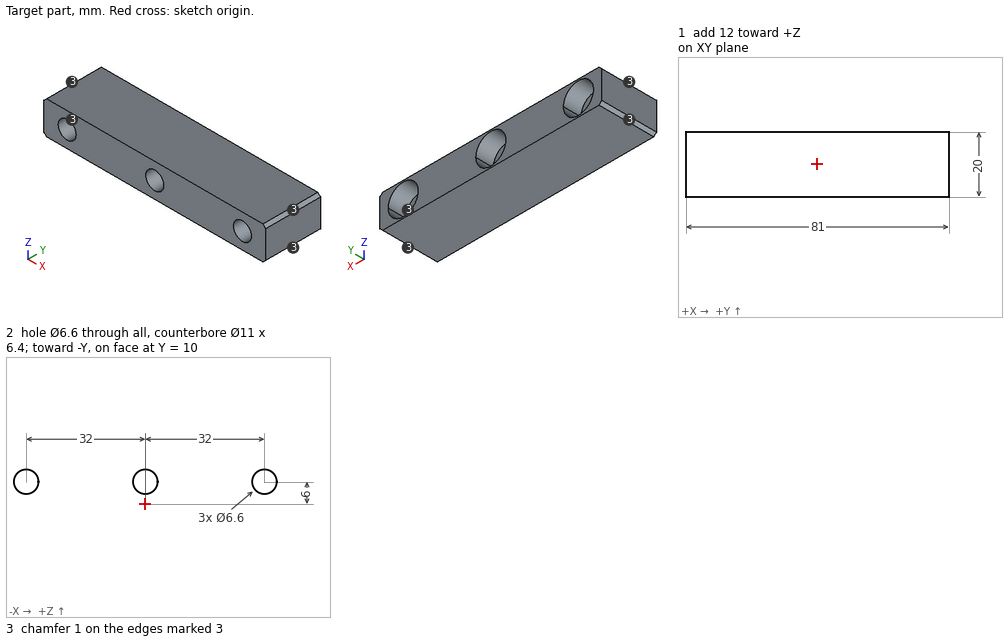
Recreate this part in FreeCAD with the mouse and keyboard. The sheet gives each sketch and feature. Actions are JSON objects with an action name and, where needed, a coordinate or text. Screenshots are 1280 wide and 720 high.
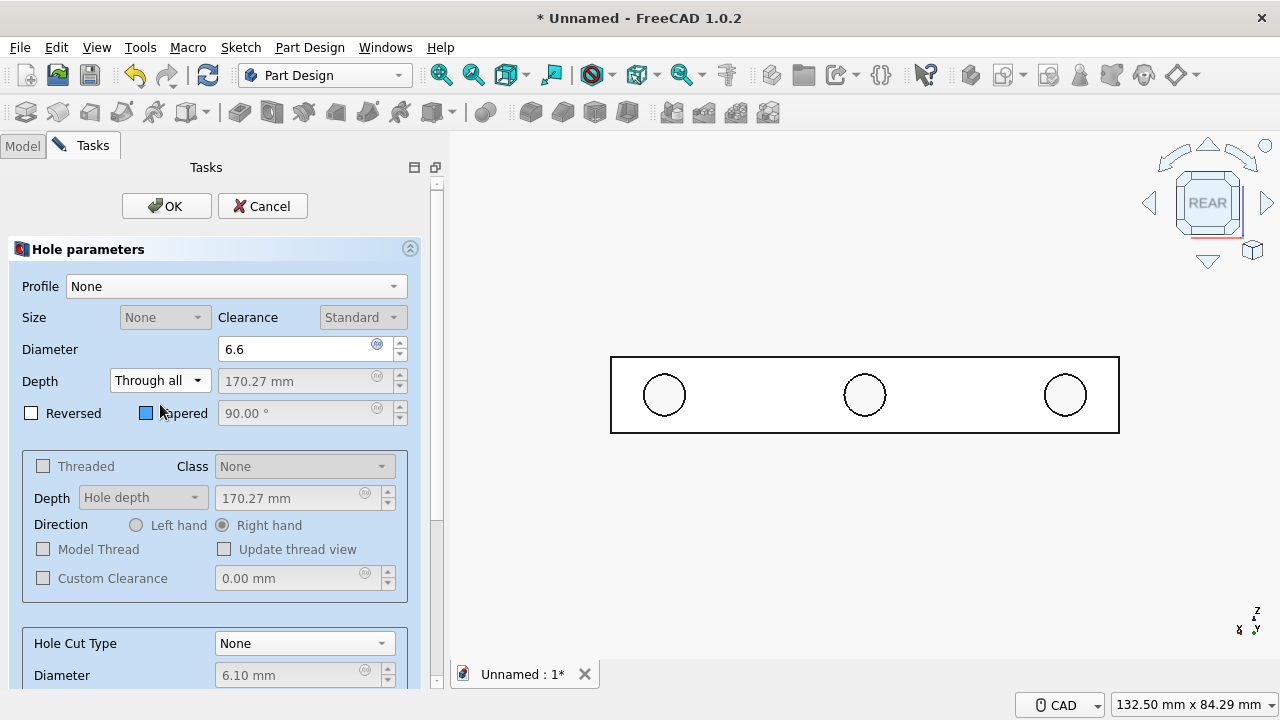
{"action": "left_click", "coordinate": [306, 644]}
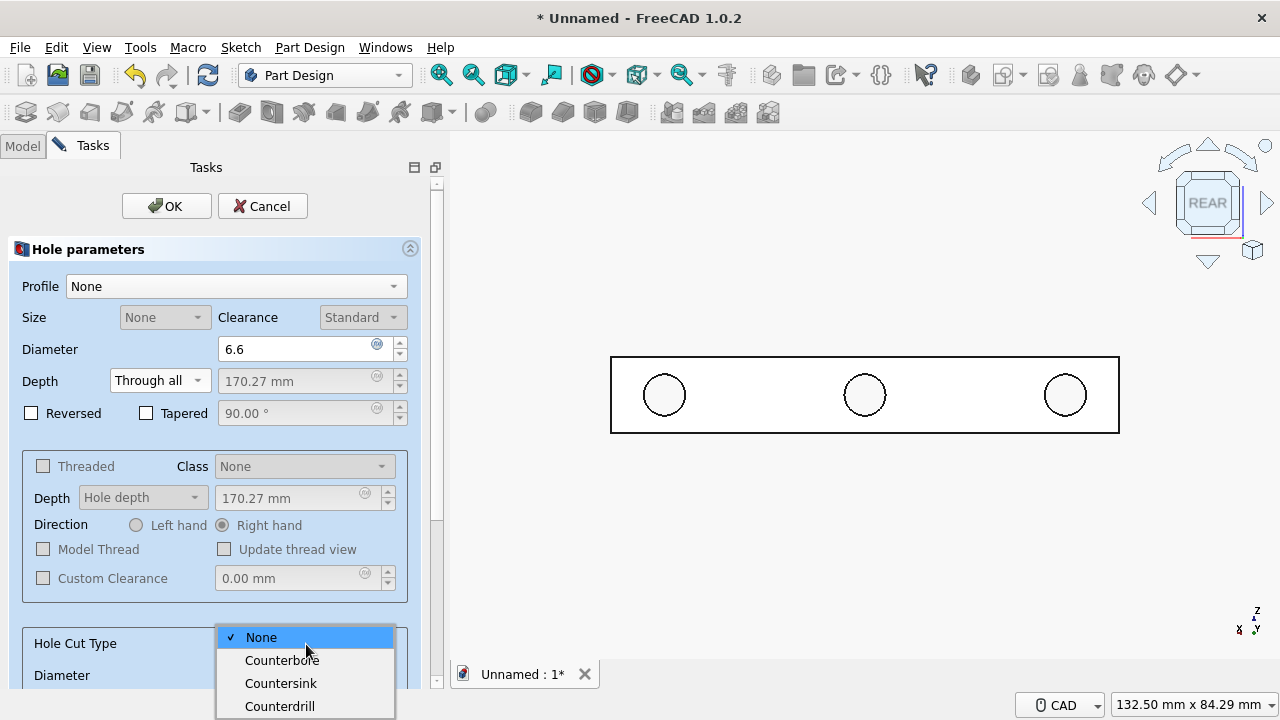
{"action": "left_click", "coordinate": [304, 660]}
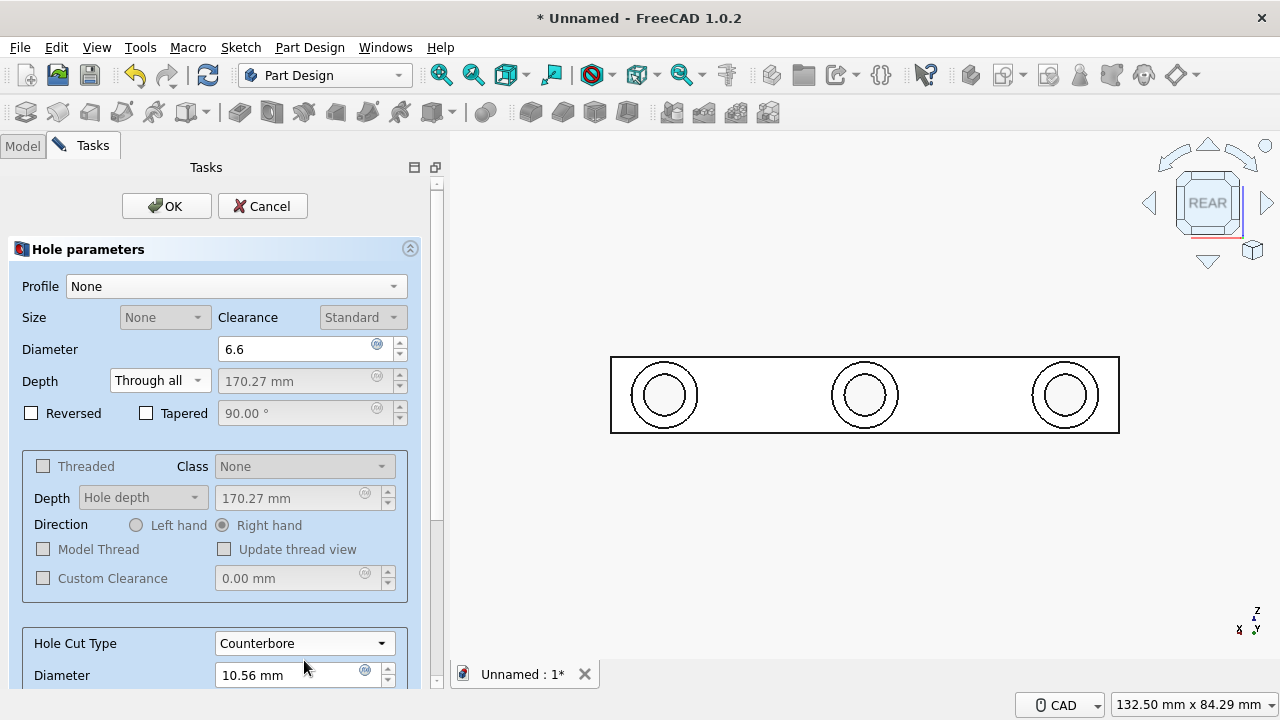
{"action": "triple_click", "coordinate": [298, 675]}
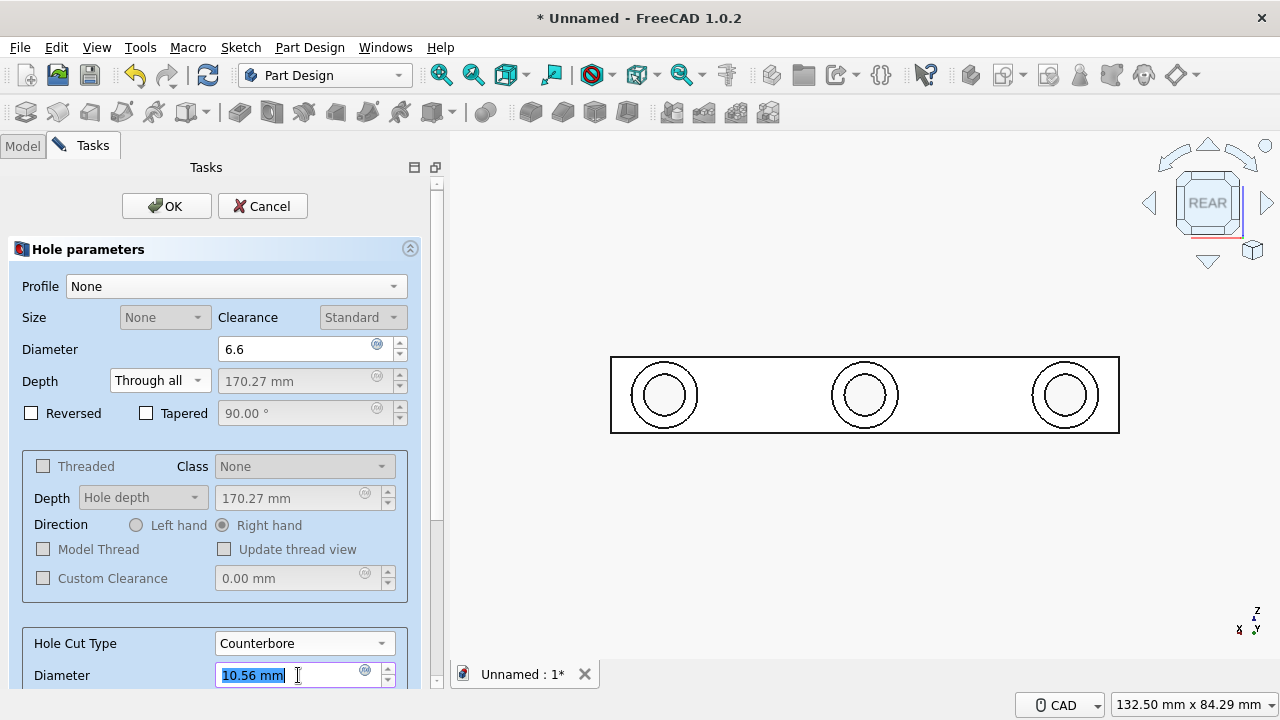
{"action": "type", "text": "11"}
{"action": "key", "text": "Tab"}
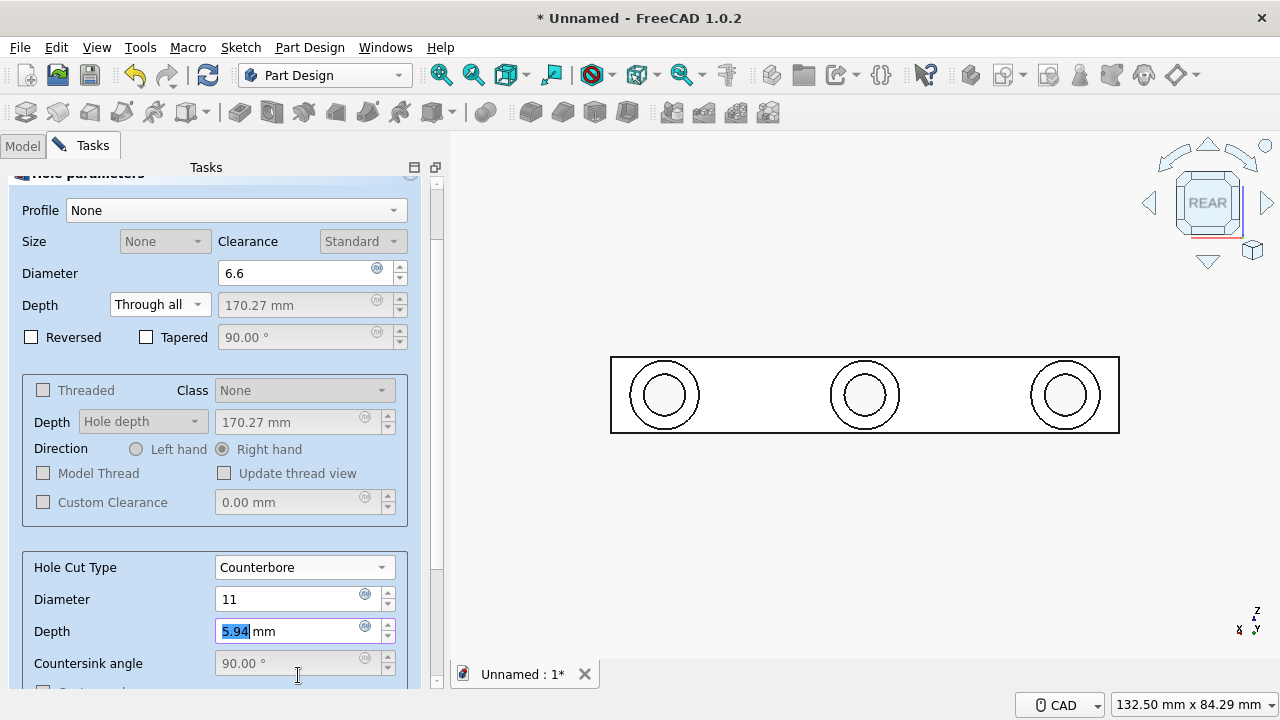
{"action": "type", "text": "6.4"}
{"action": "key", "text": "Tab"}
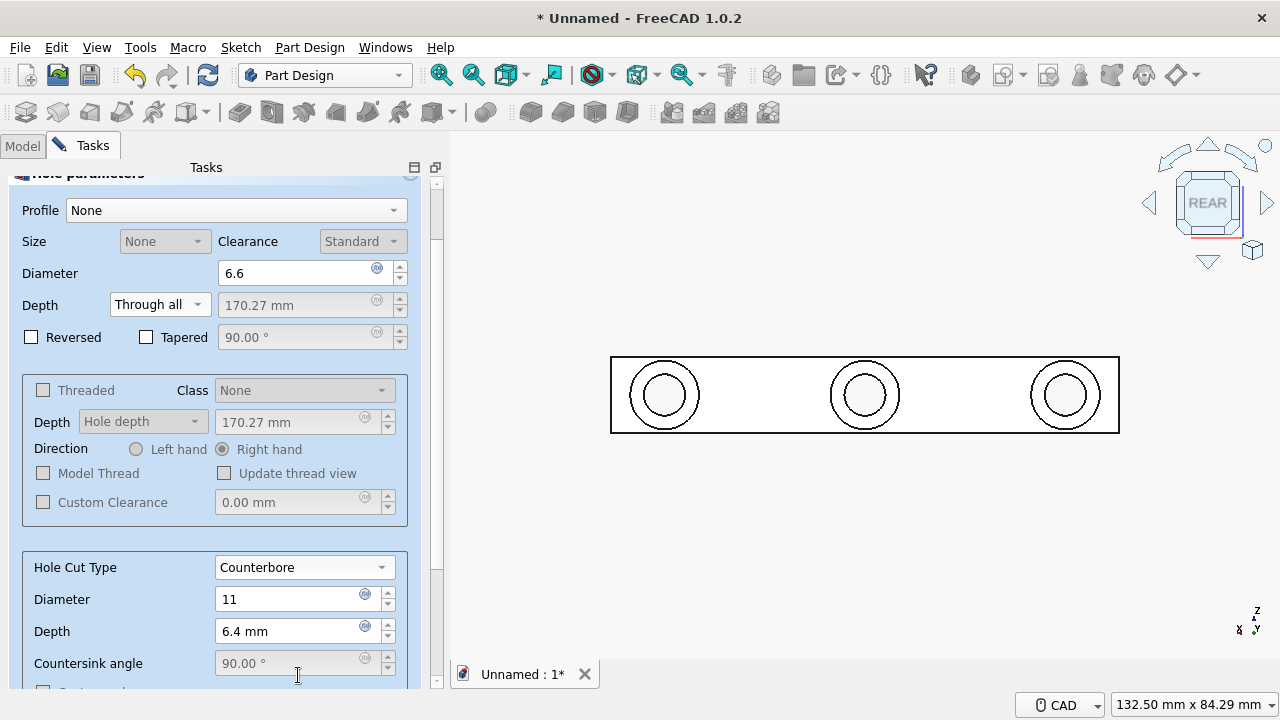
{"action": "scroll", "coordinate": [437, 432], "scroll_direction": "up", "scroll_amount": 3}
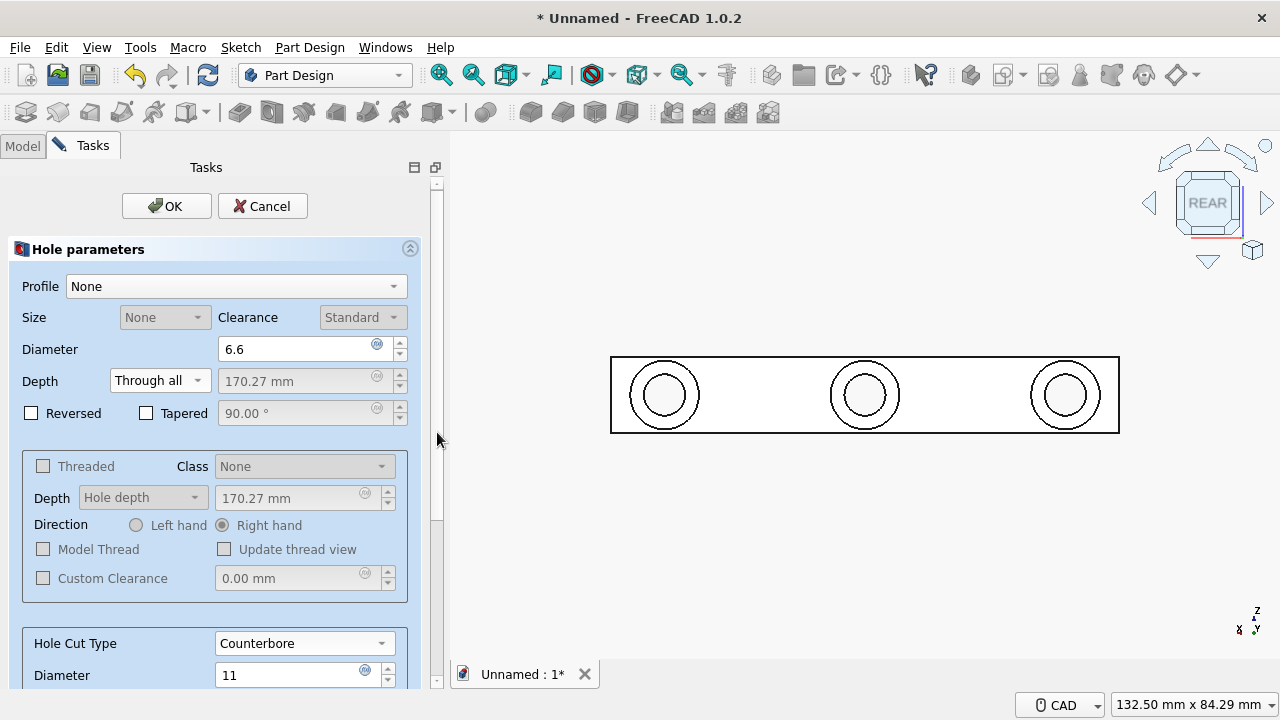
{"action": "left_click", "coordinate": [167, 206]}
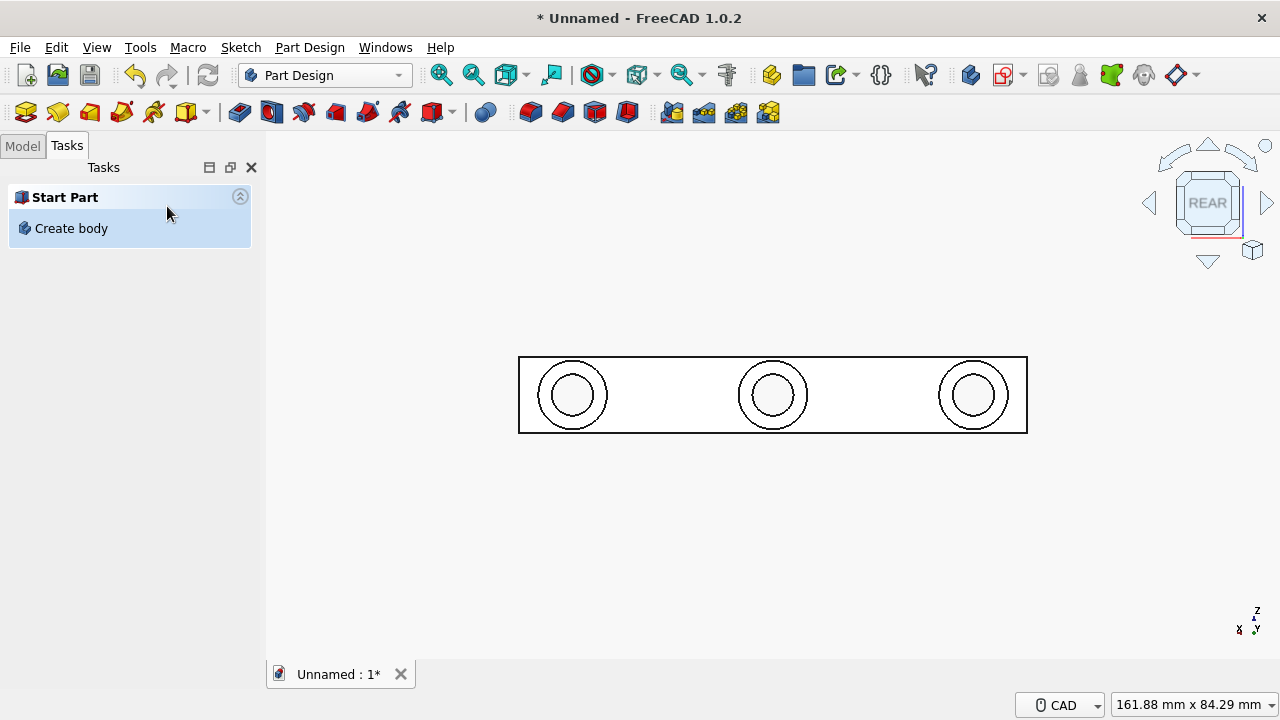
{"action": "key", "text": "0"}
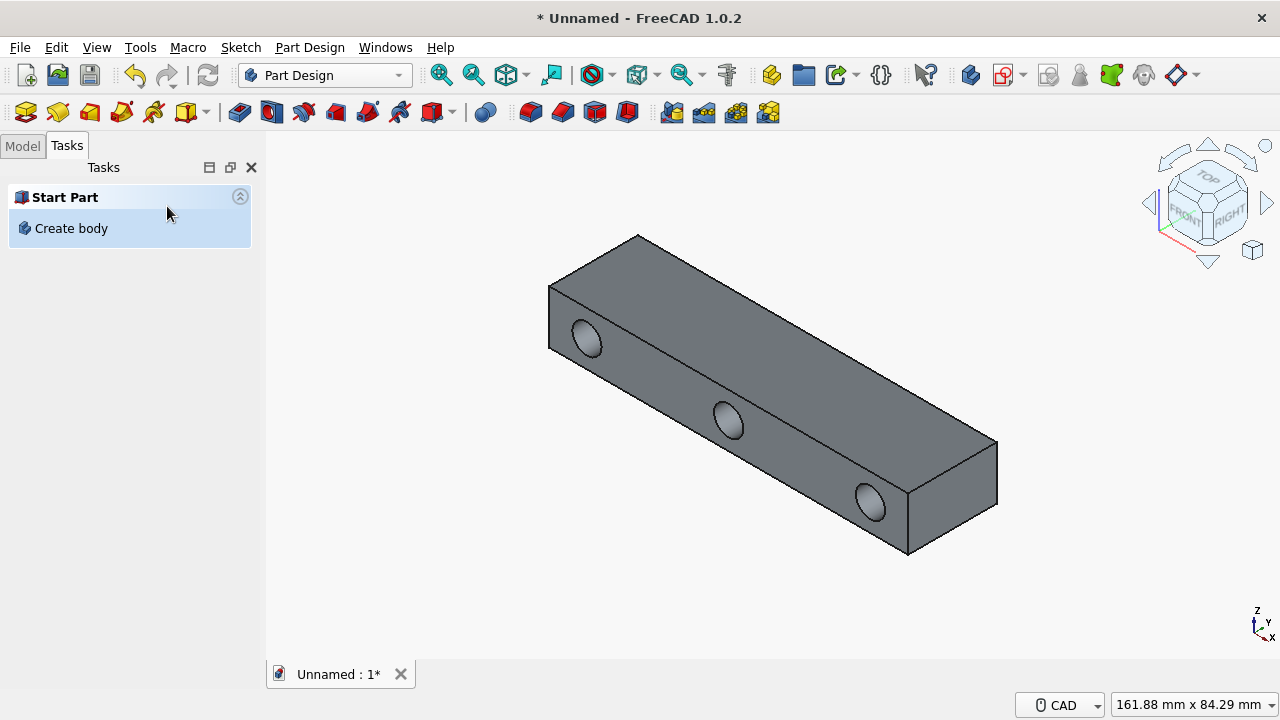
{"action": "left_click", "coordinate": [952, 467]}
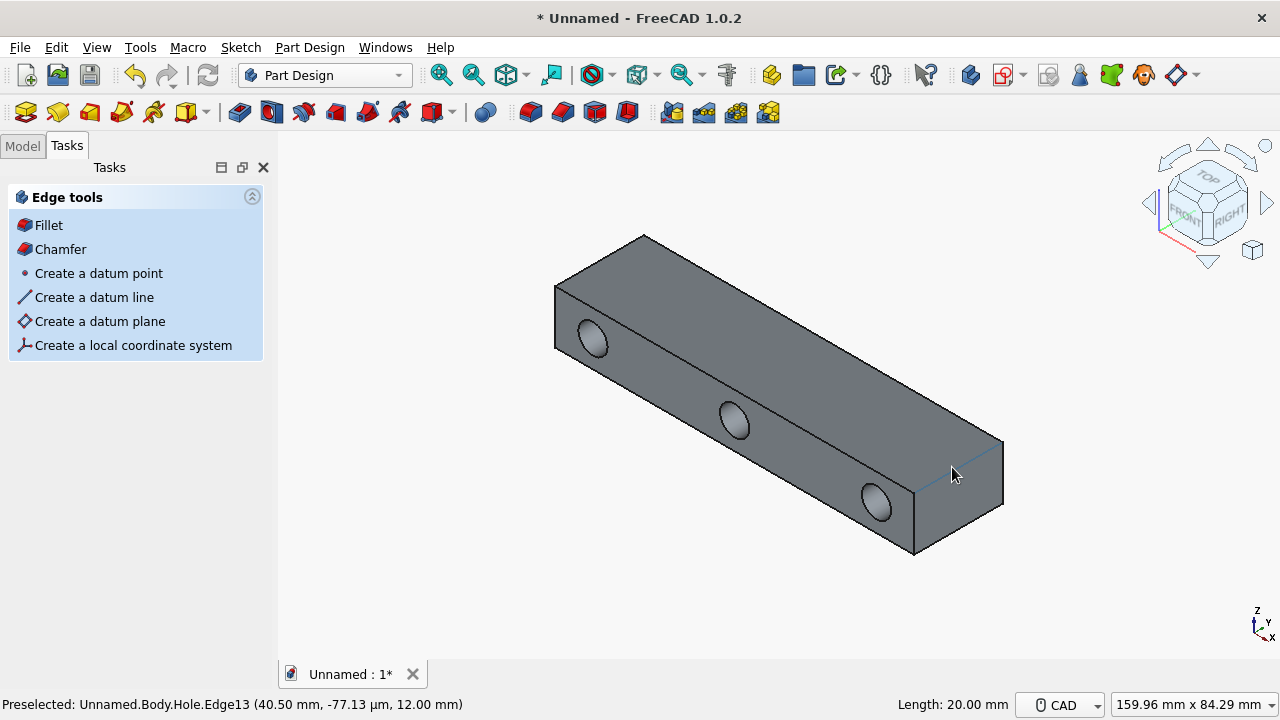
{"action": "key", "text": "2"}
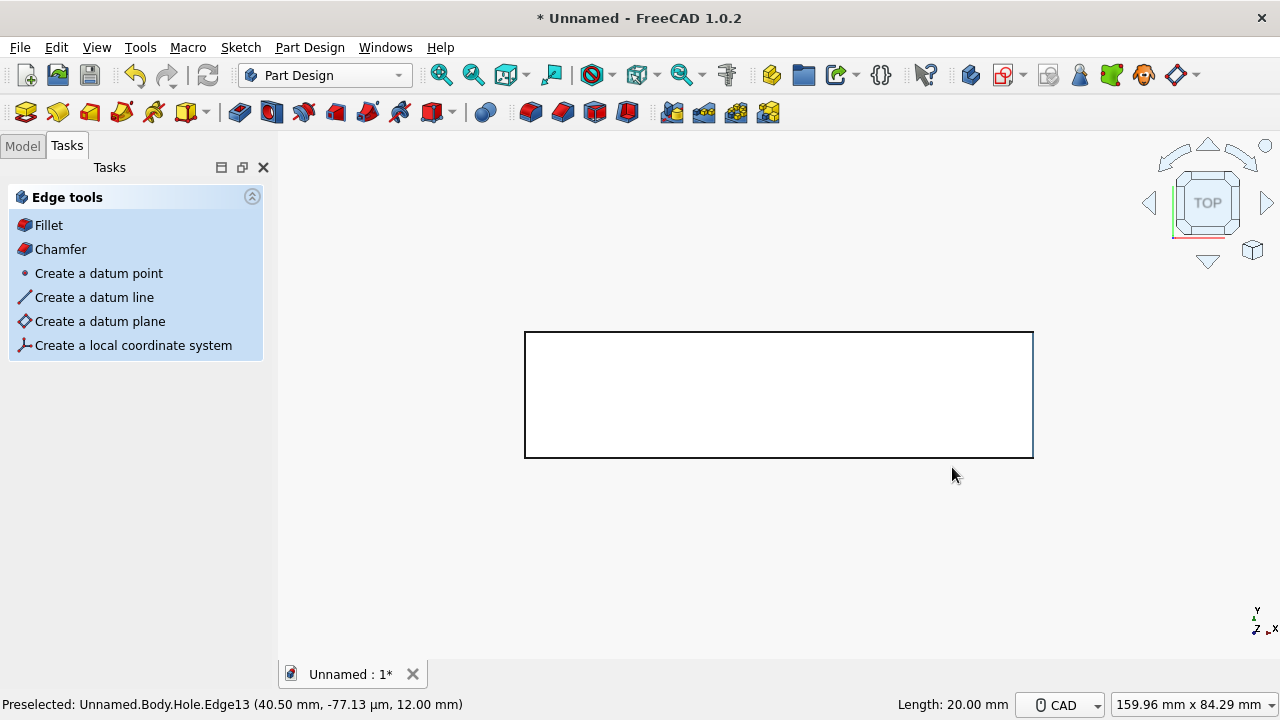
{"action": "left_click", "coordinate": [525, 394], "text": "ctrl"}